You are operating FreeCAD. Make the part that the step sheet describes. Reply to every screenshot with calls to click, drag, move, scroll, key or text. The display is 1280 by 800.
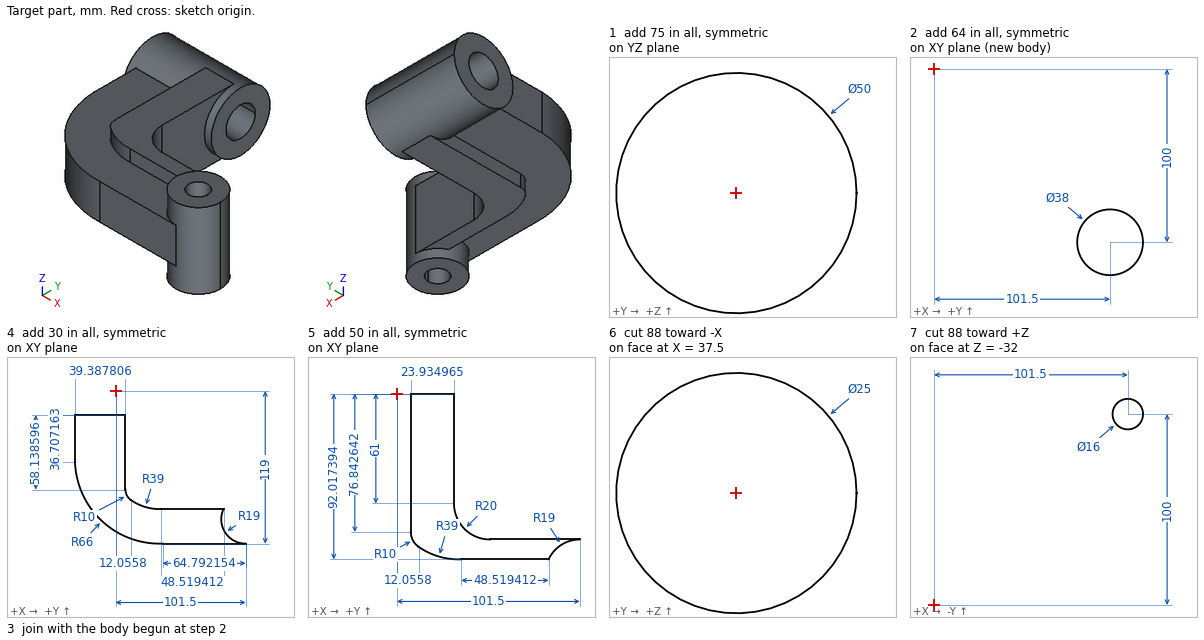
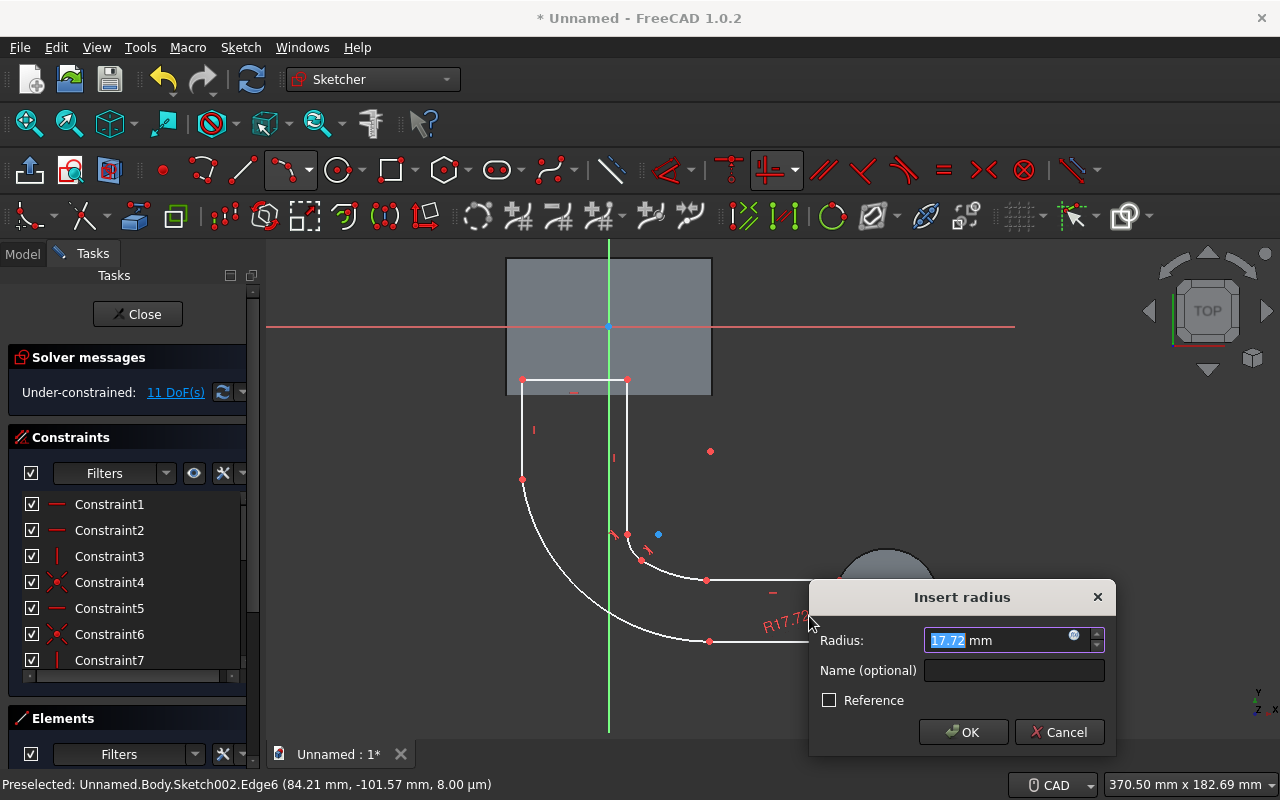
text(19)
key(Return)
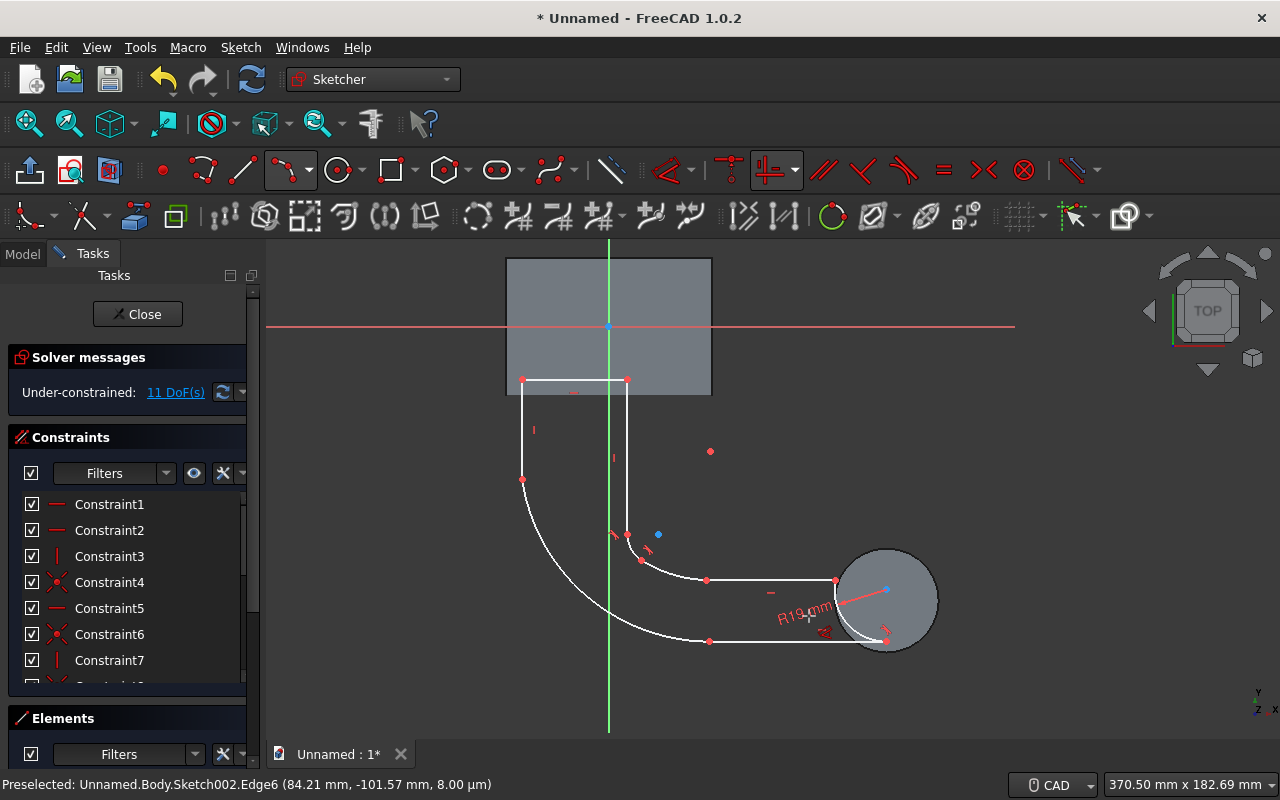
click(660, 570)
click(648, 599)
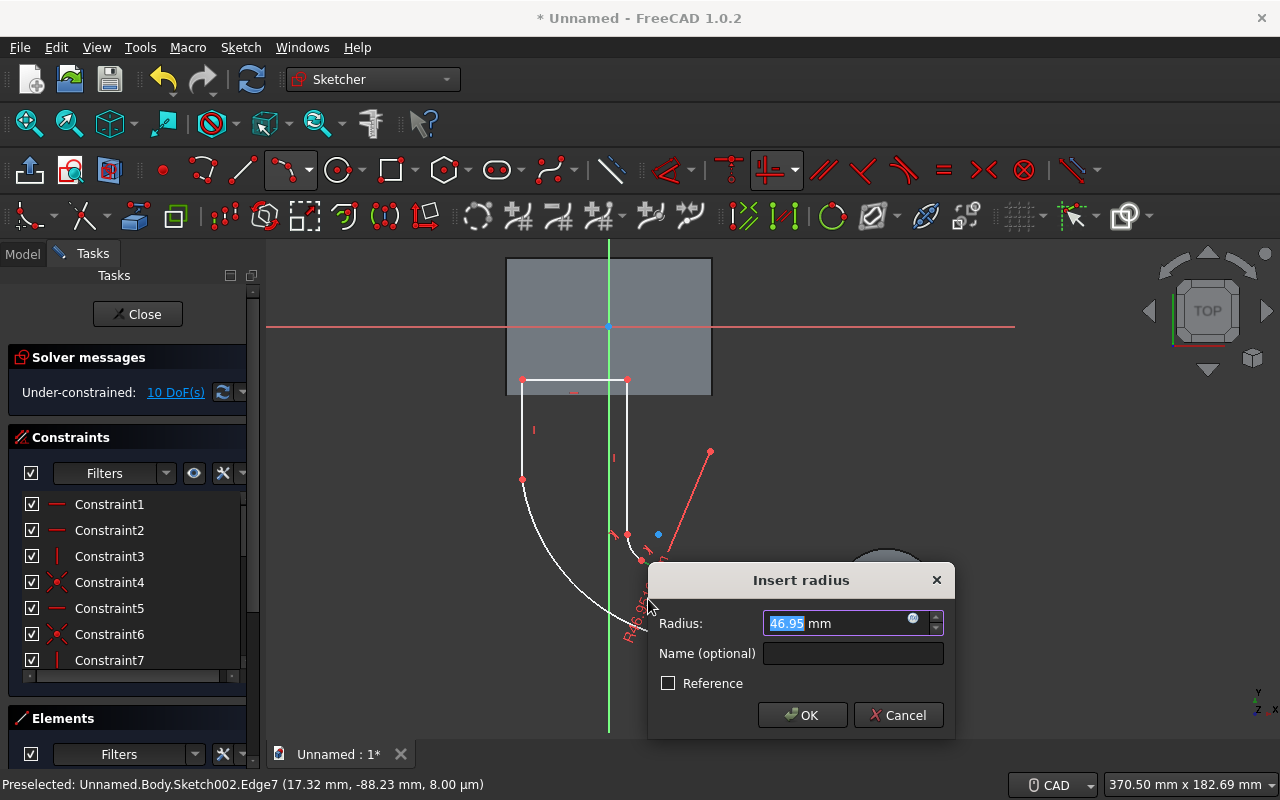
text(39)
key(Return)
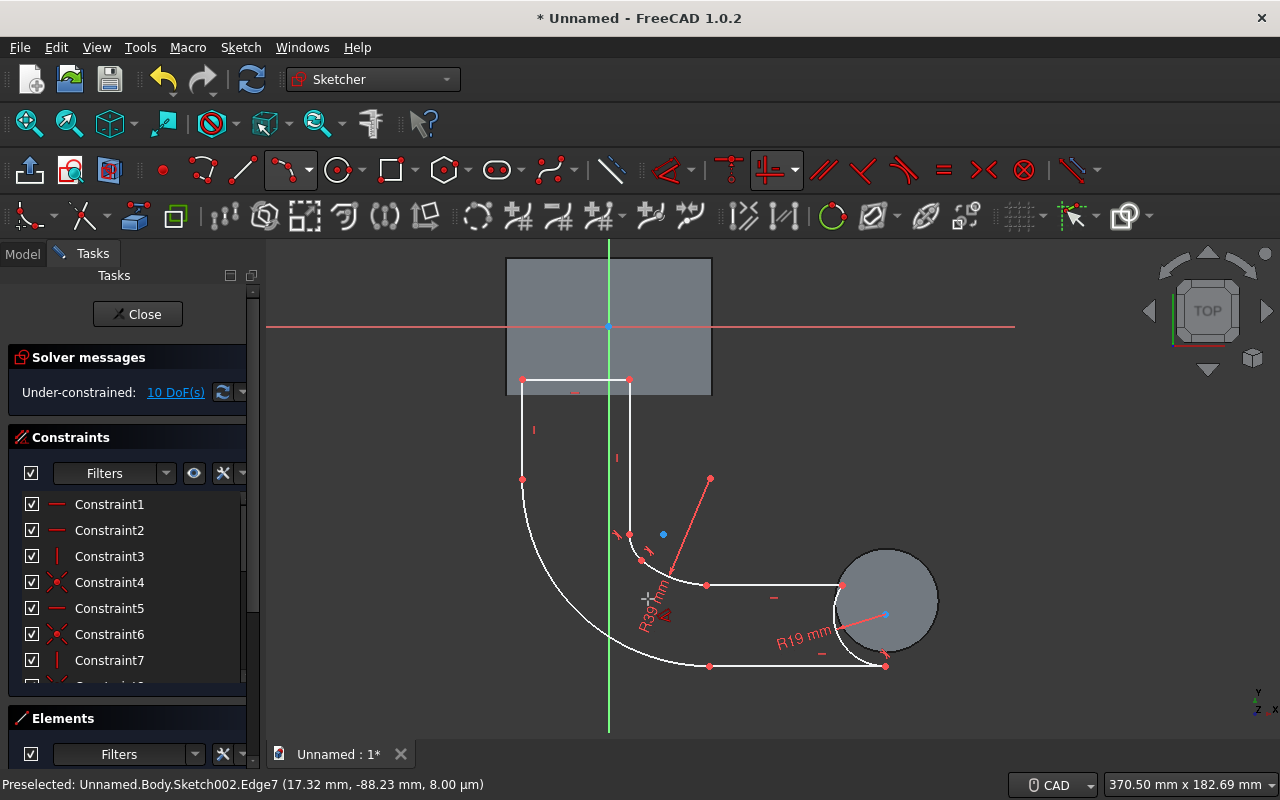
scroll(633, 549, up, 2)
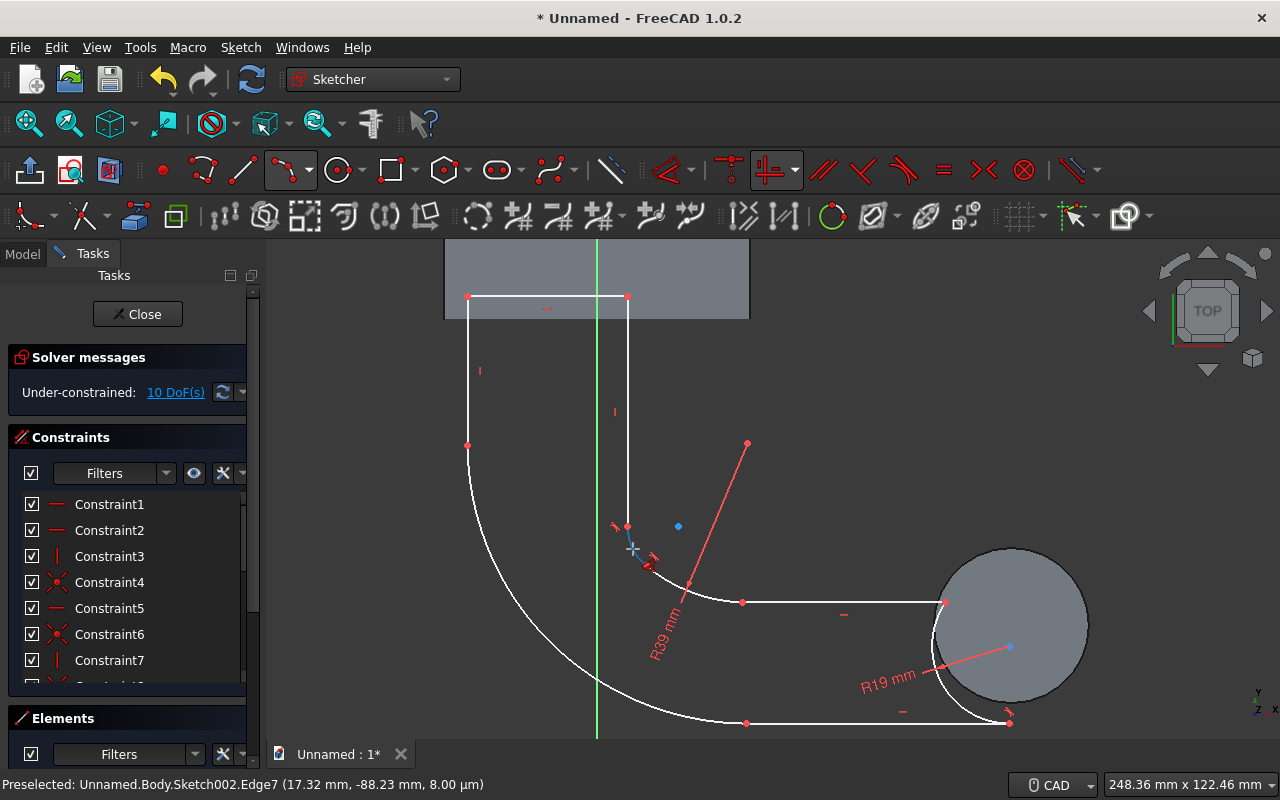
click(633, 548)
click(630, 593)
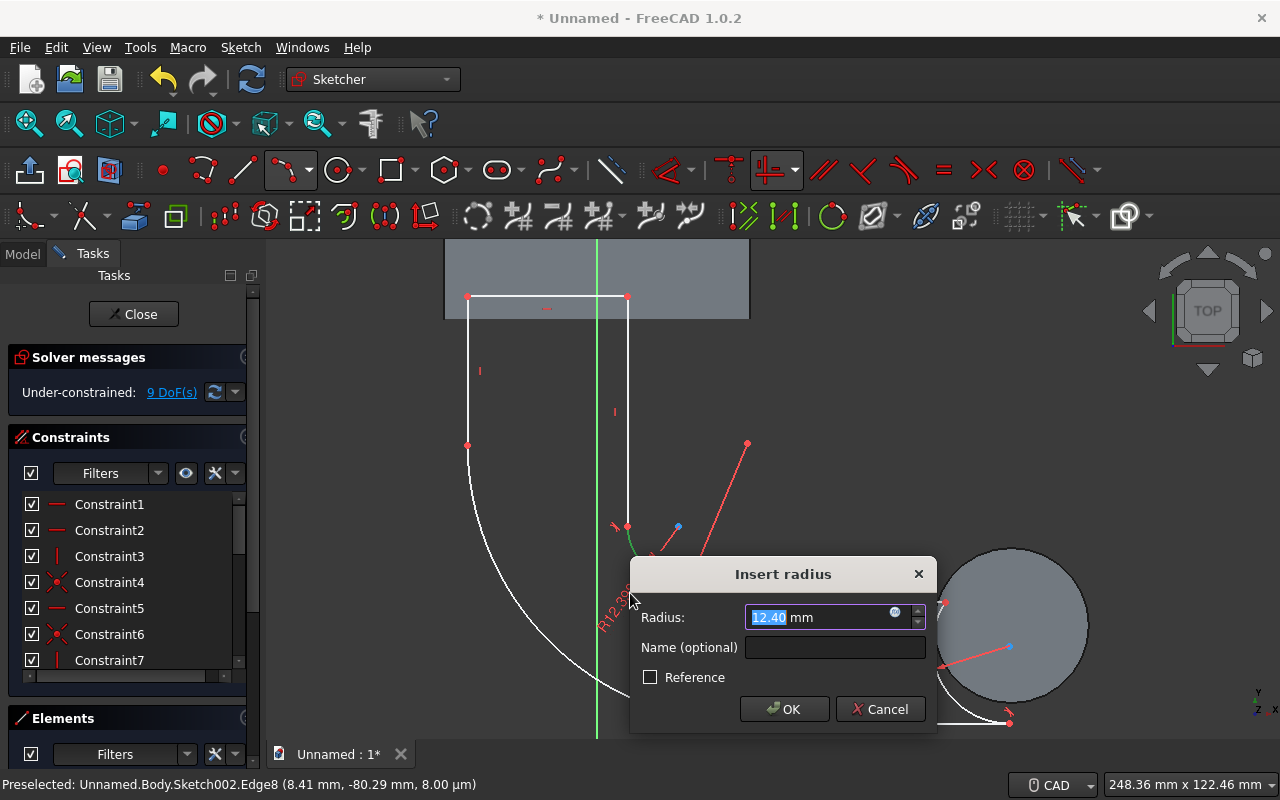
text(10)
key(Return)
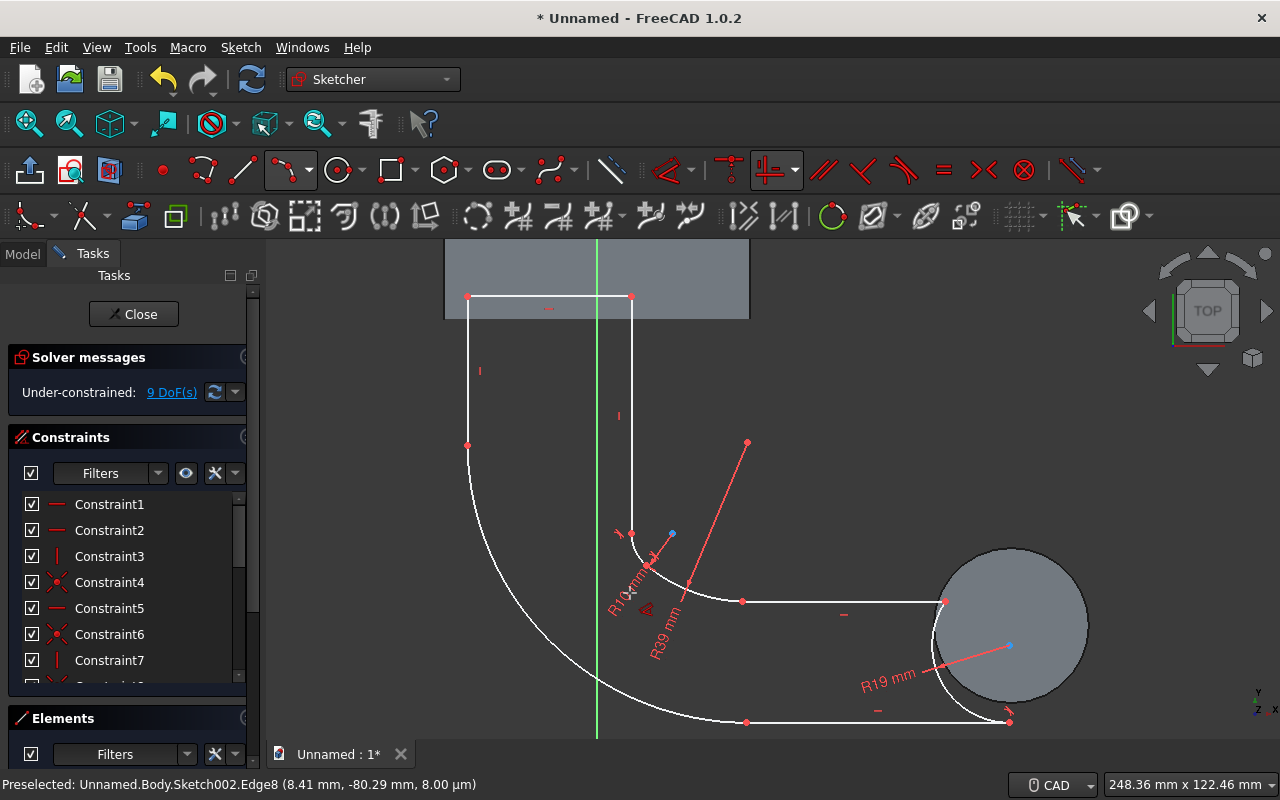
click(499, 571)
click(471, 586)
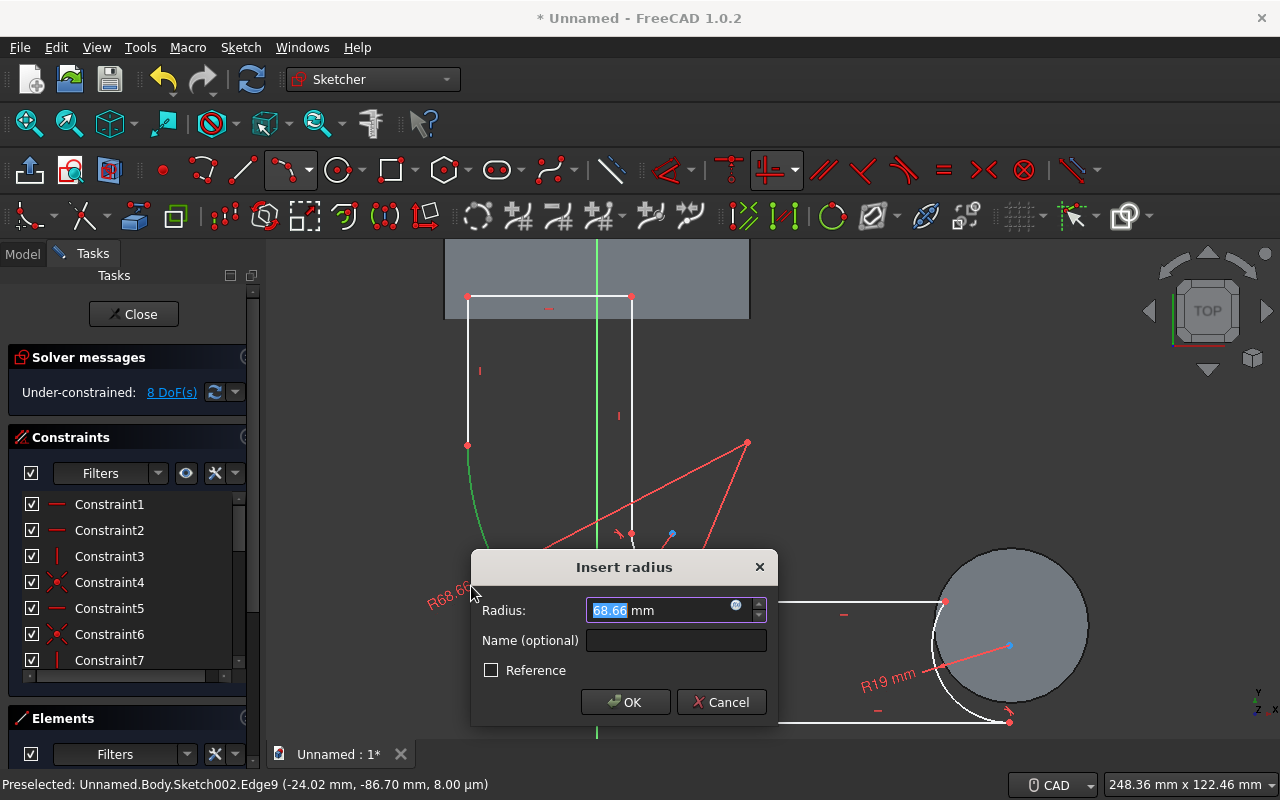
text(66)
key(Return)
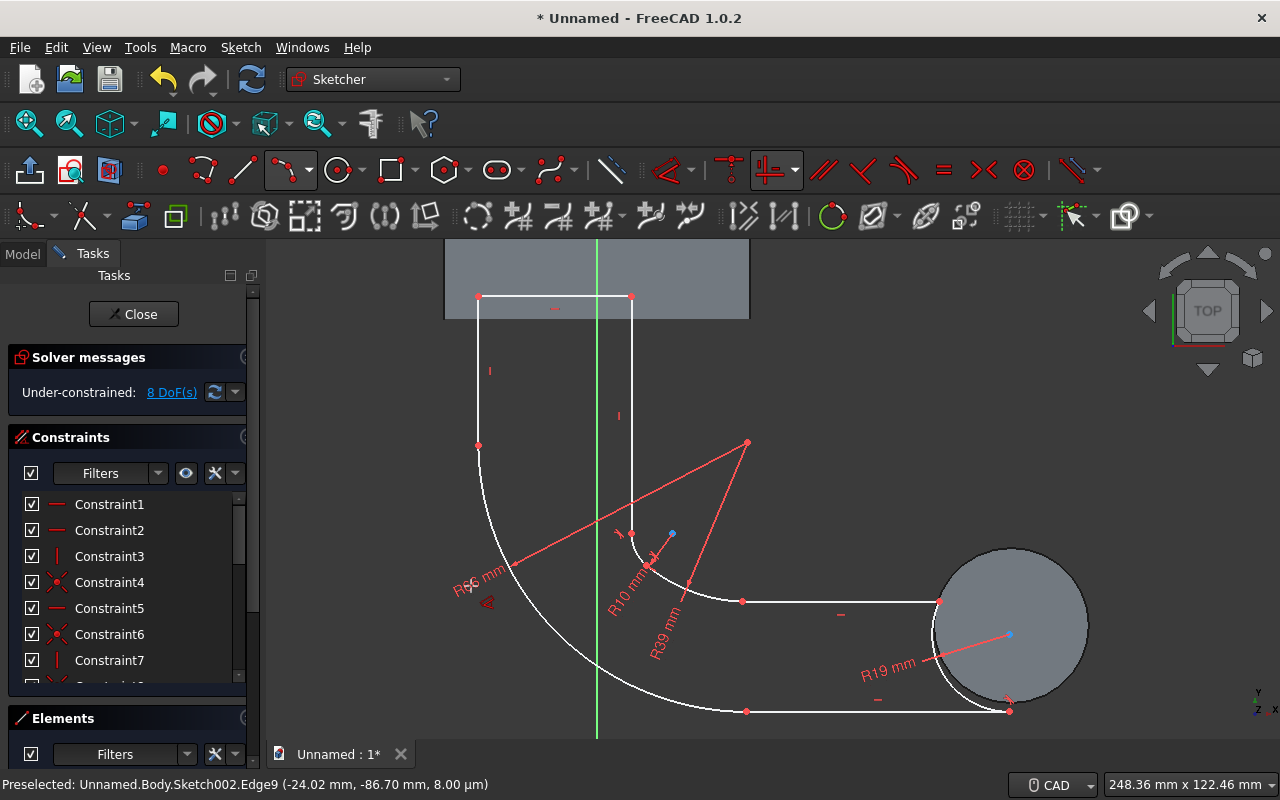
scroll(633, 548, down, 2)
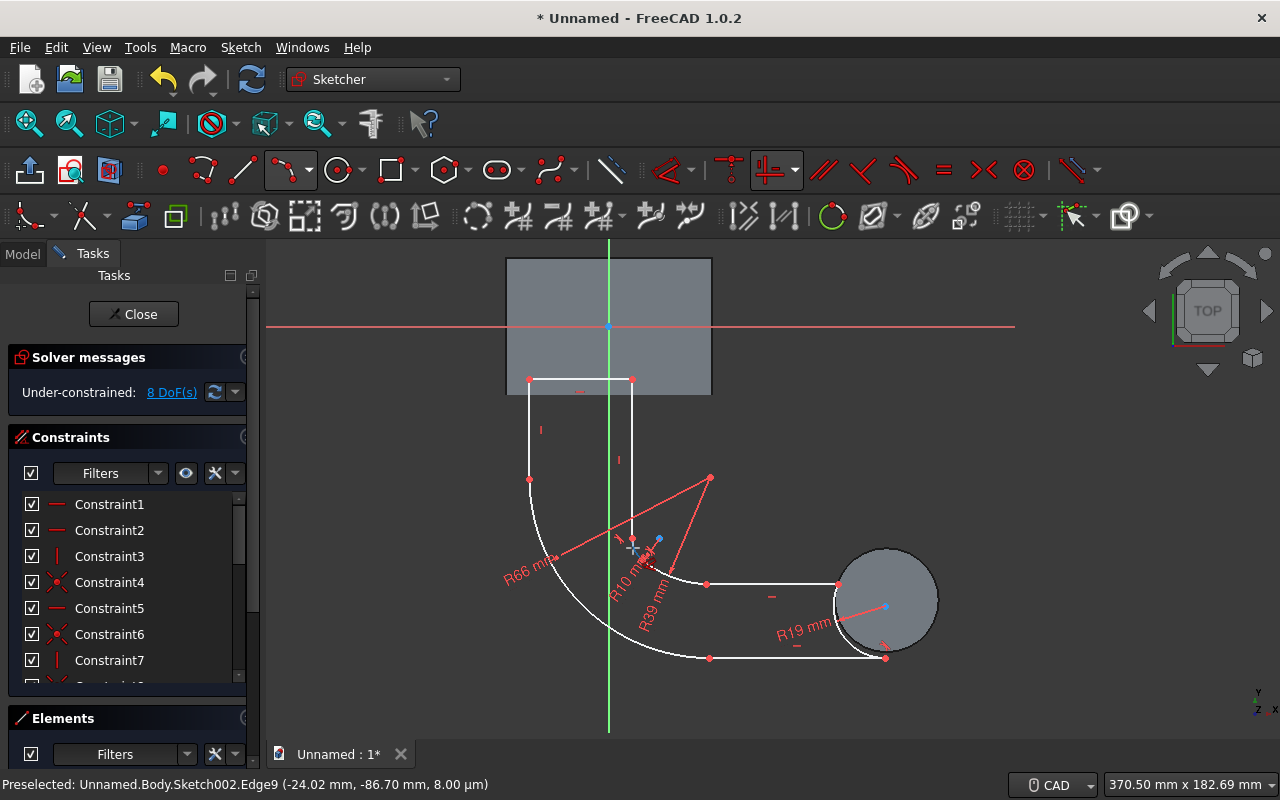
click(709, 658)
click(575, 492)